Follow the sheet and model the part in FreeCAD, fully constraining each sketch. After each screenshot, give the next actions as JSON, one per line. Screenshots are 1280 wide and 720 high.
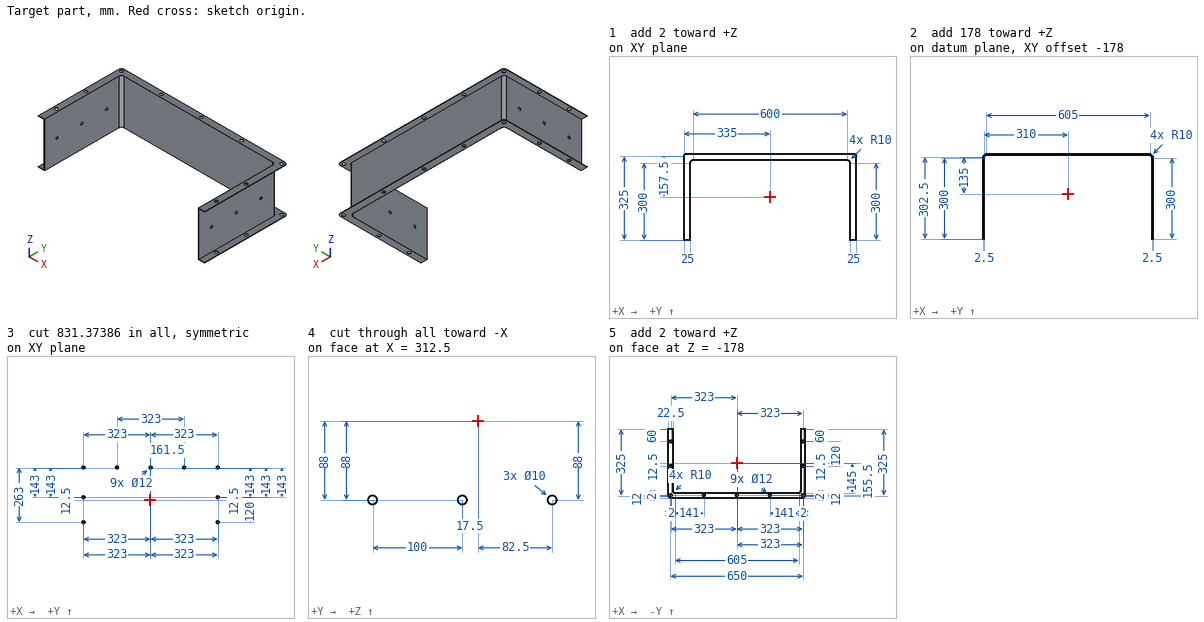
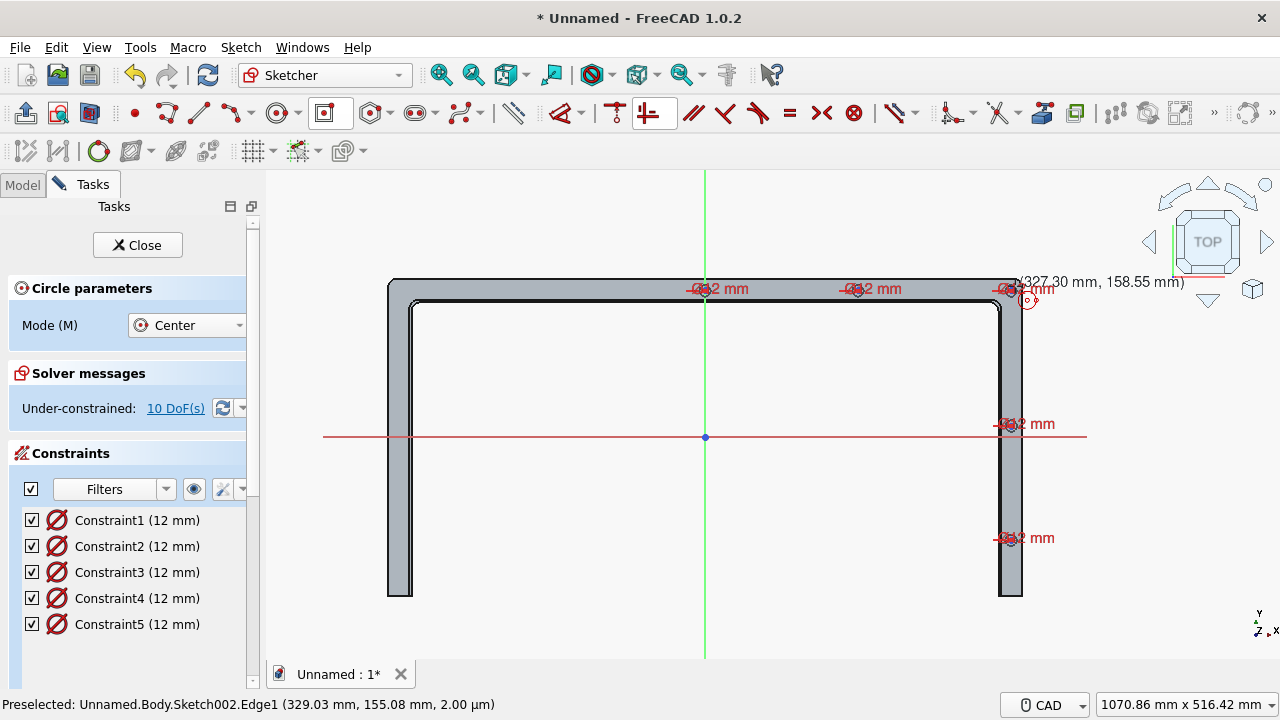
{"action": "scroll", "coordinate": [399, 290], "scroll_direction": "up", "scroll_amount": 7}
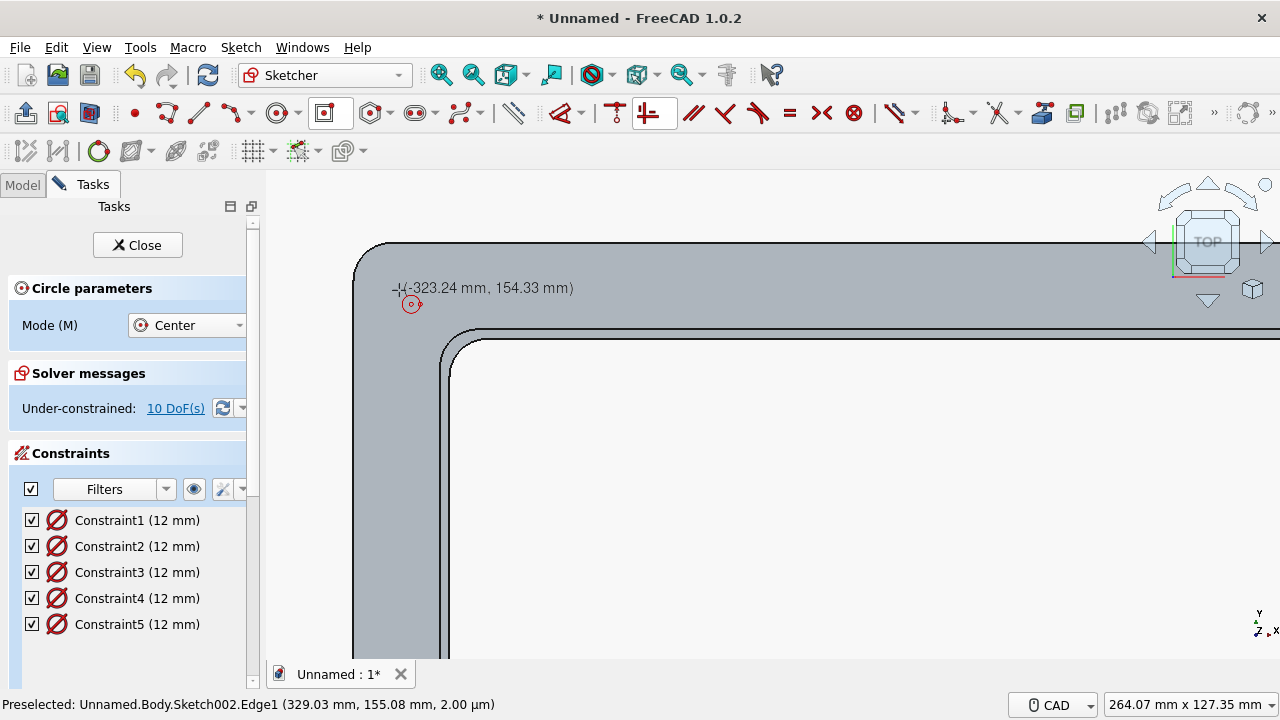
{"action": "scroll", "coordinate": [398, 290], "scroll_direction": "down", "scroll_amount": 7}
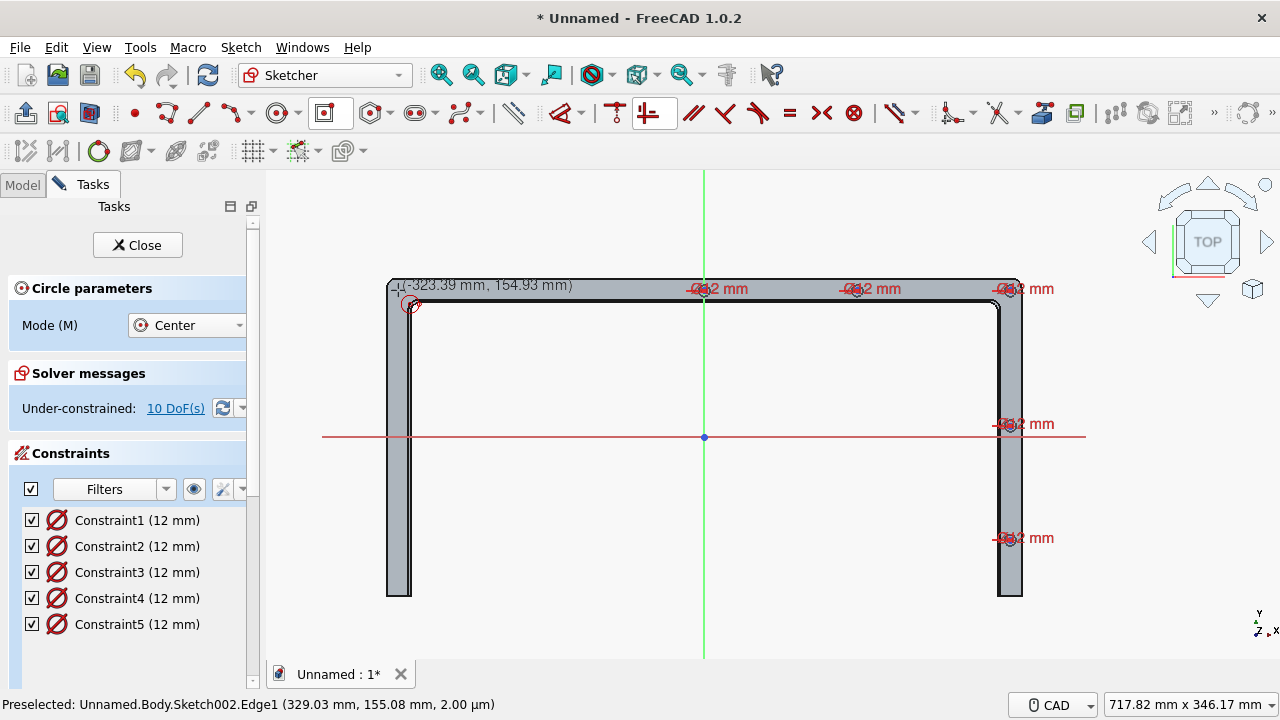
{"action": "left_click", "coordinate": [398, 290]}
{"action": "mouse_move", "coordinate": [402, 286]}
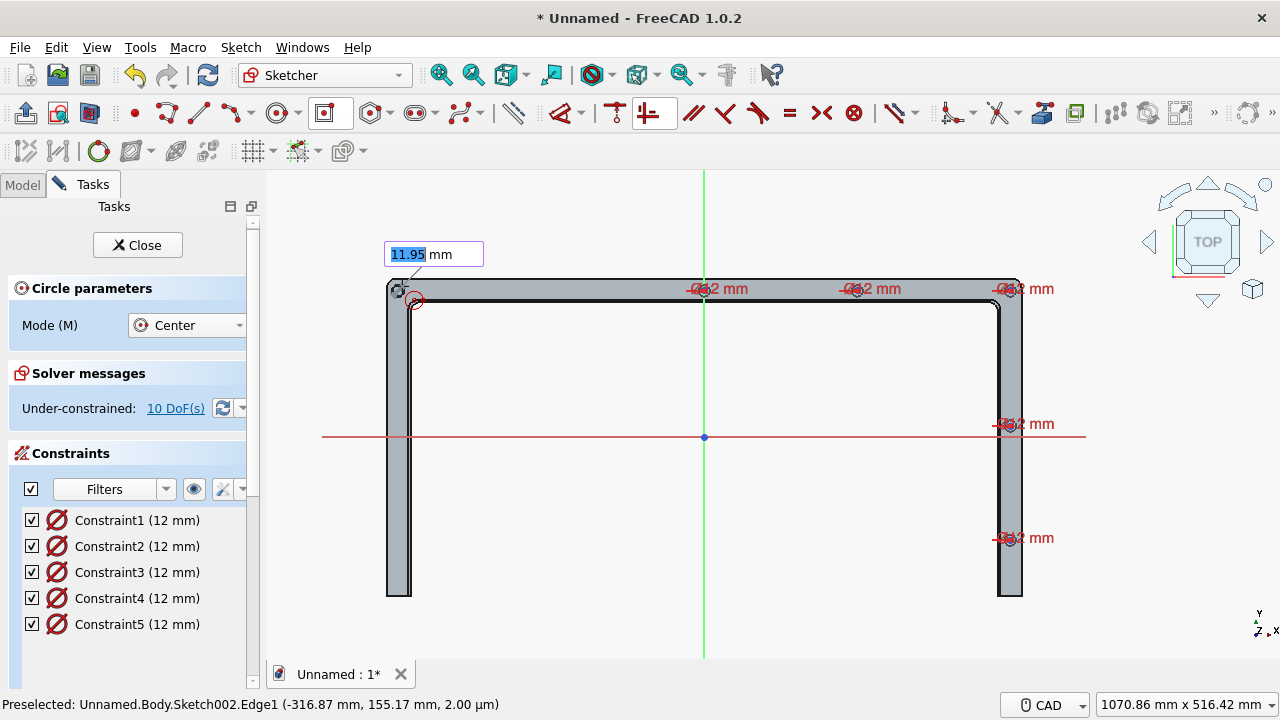
{"action": "type", "text": "12"}
{"action": "key", "text": "Return"}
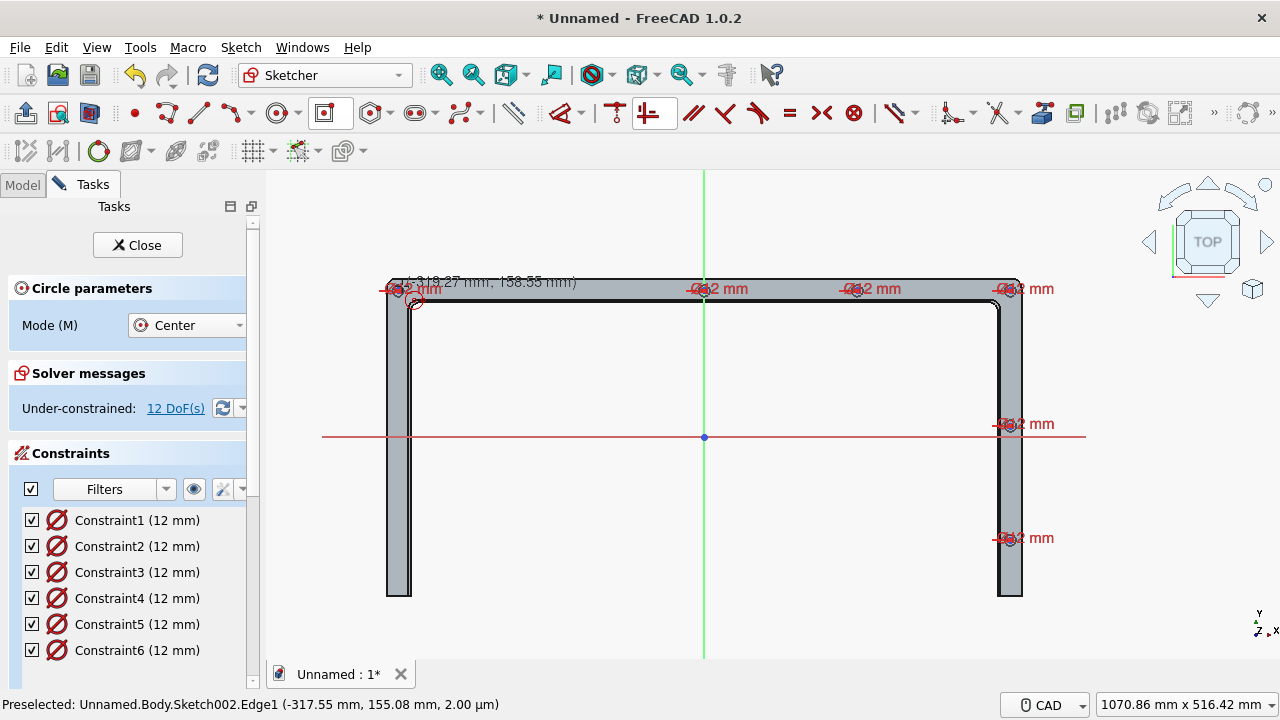
{"action": "scroll", "coordinate": [398, 539], "scroll_direction": "up", "scroll_amount": 7}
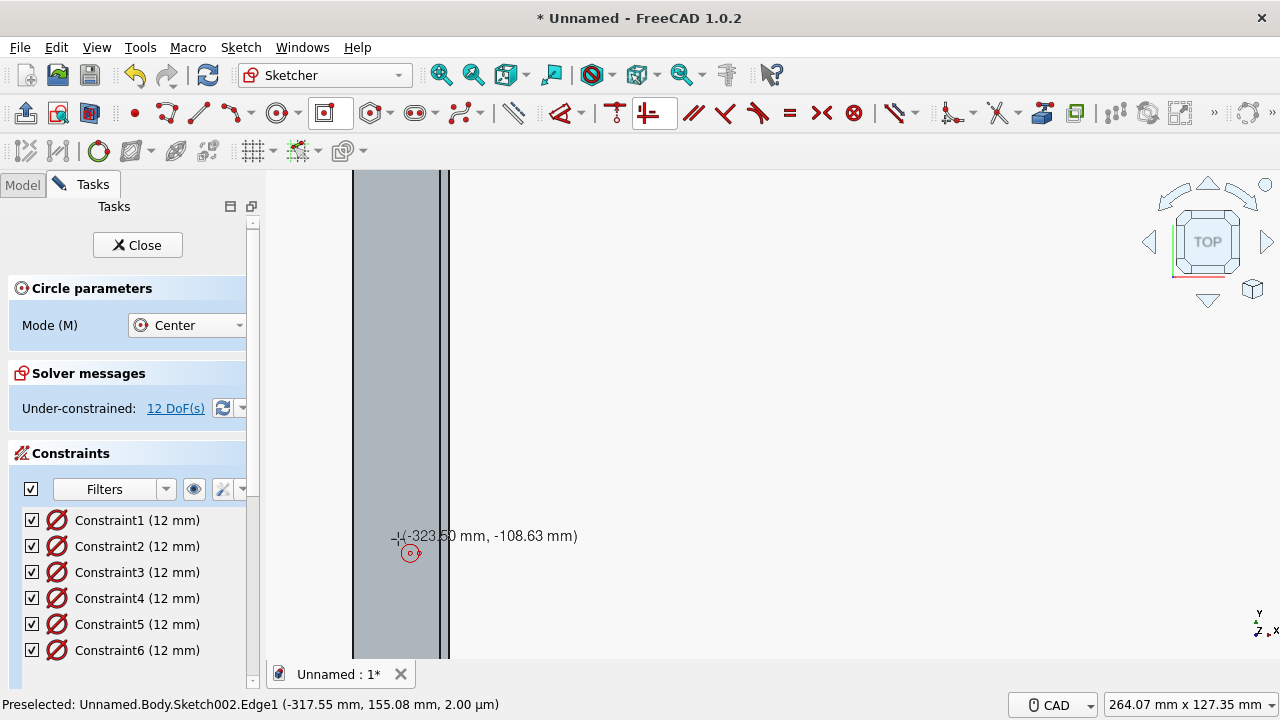
{"action": "scroll", "coordinate": [398, 540], "scroll_direction": "down", "scroll_amount": 7}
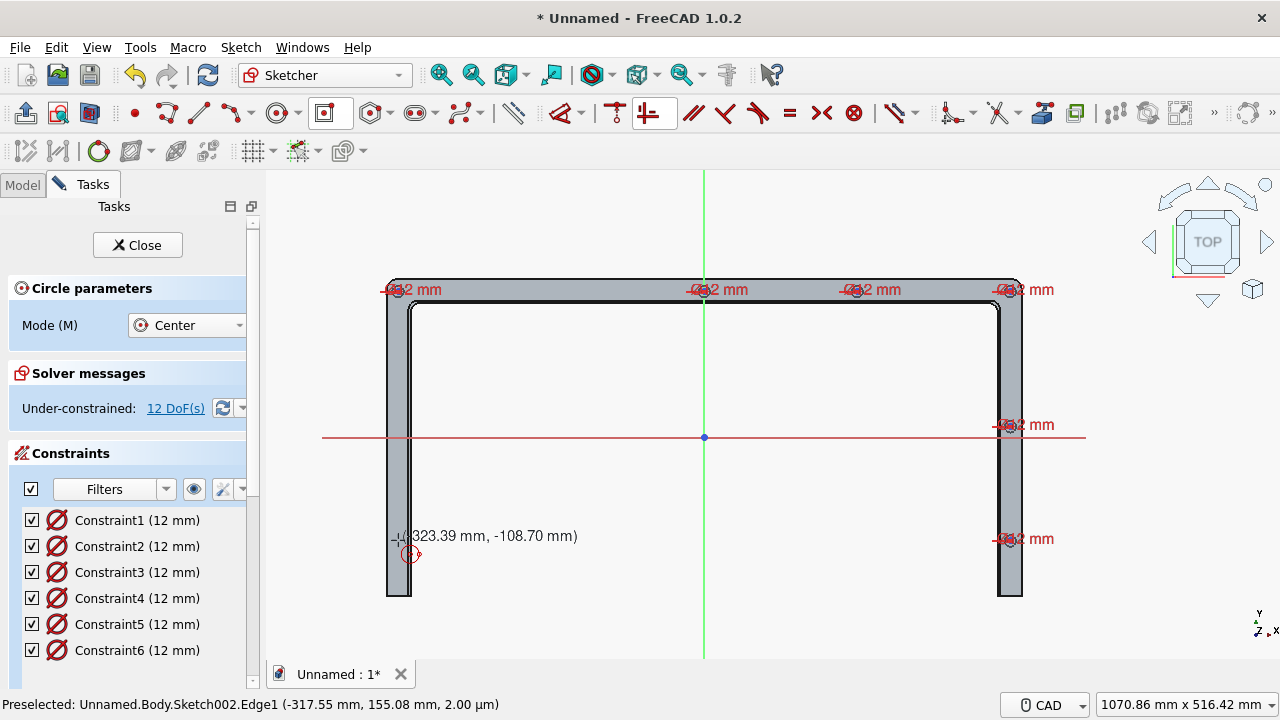
{"action": "left_click", "coordinate": [398, 540]}
{"action": "mouse_move", "coordinate": [402, 536]}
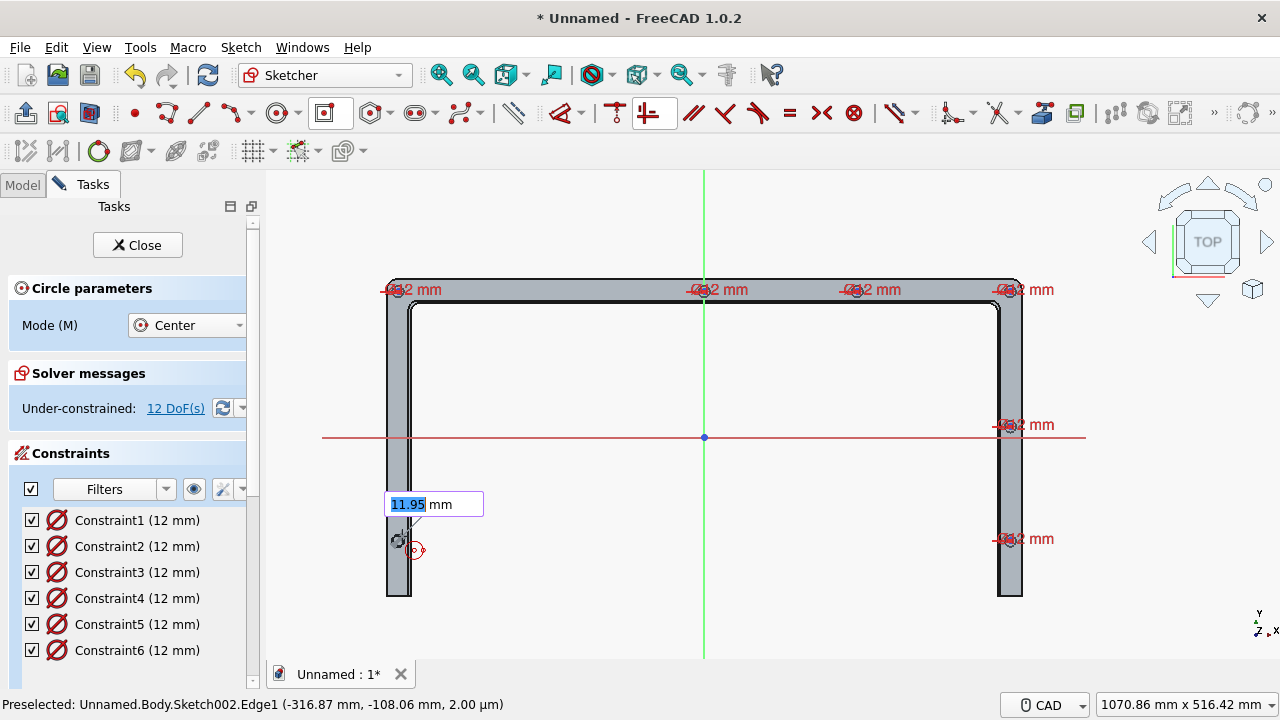
{"action": "type", "text": "12"}
{"action": "key", "text": "Return"}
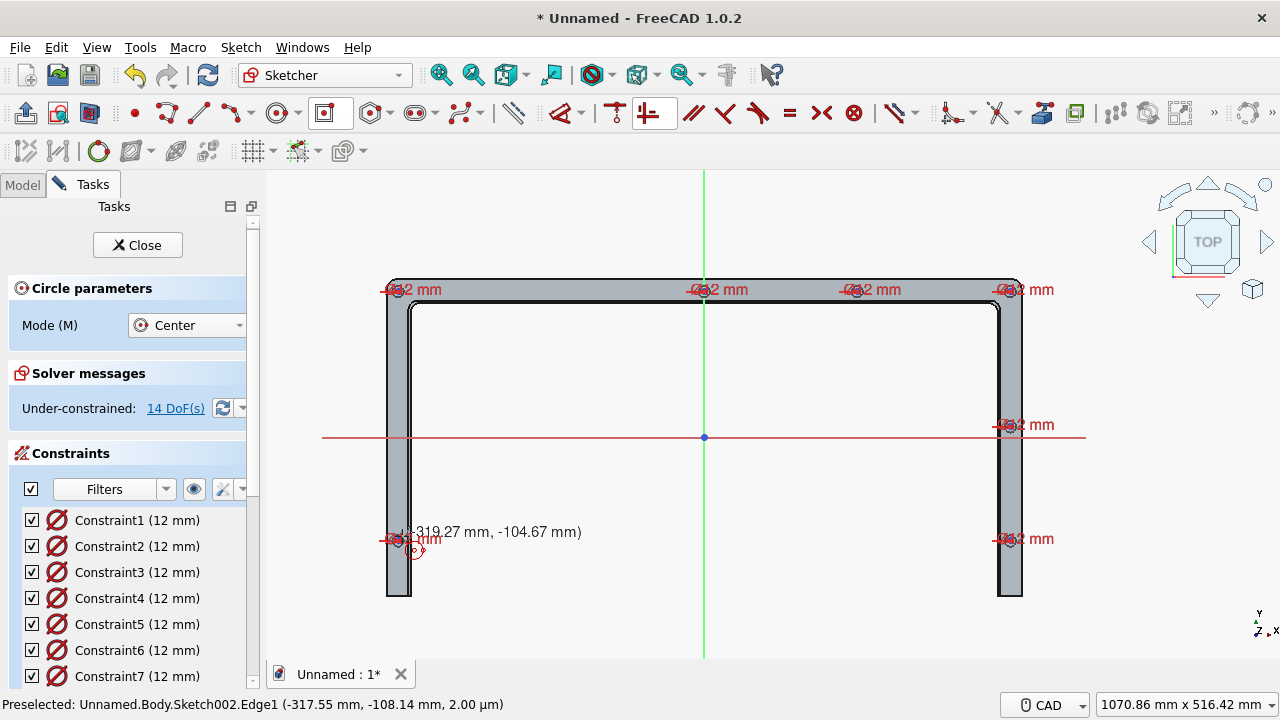
{"action": "scroll", "coordinate": [398, 426], "scroll_direction": "up", "scroll_amount": 7}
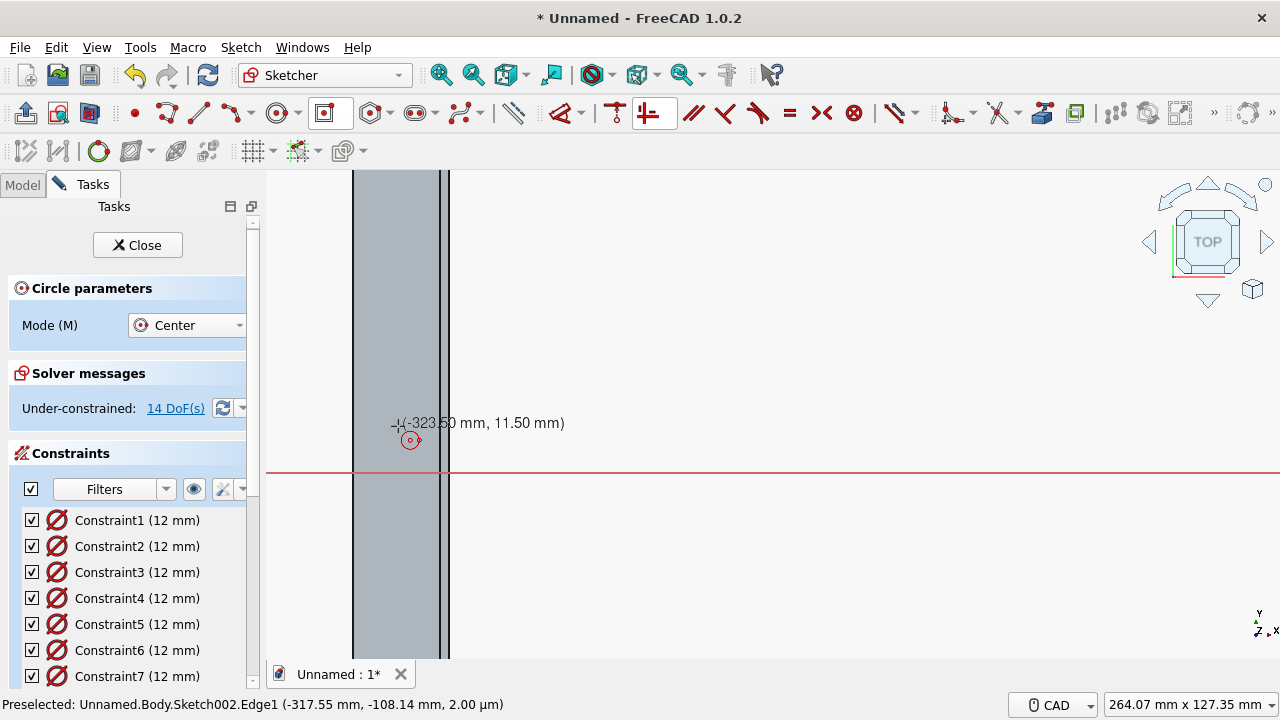
{"action": "scroll", "coordinate": [398, 426], "scroll_direction": "down", "scroll_amount": 7}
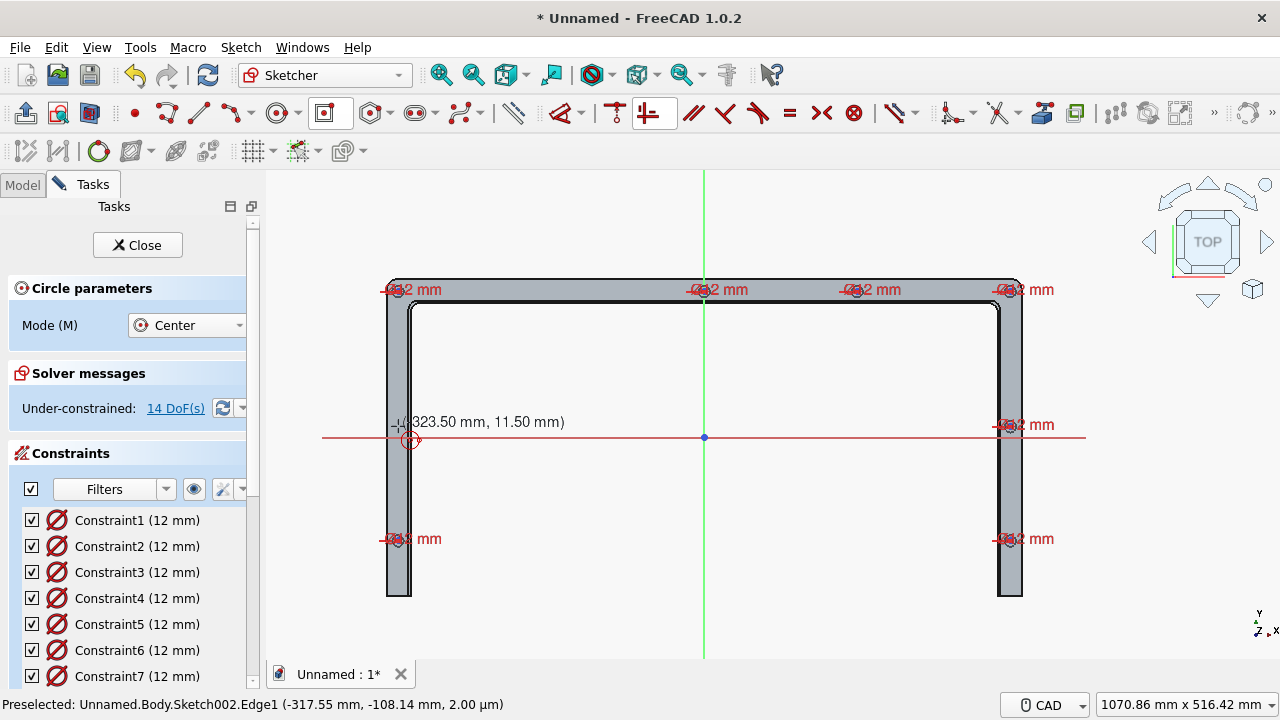
{"action": "scroll", "coordinate": [398, 426], "scroll_direction": "up", "scroll_amount": 2}